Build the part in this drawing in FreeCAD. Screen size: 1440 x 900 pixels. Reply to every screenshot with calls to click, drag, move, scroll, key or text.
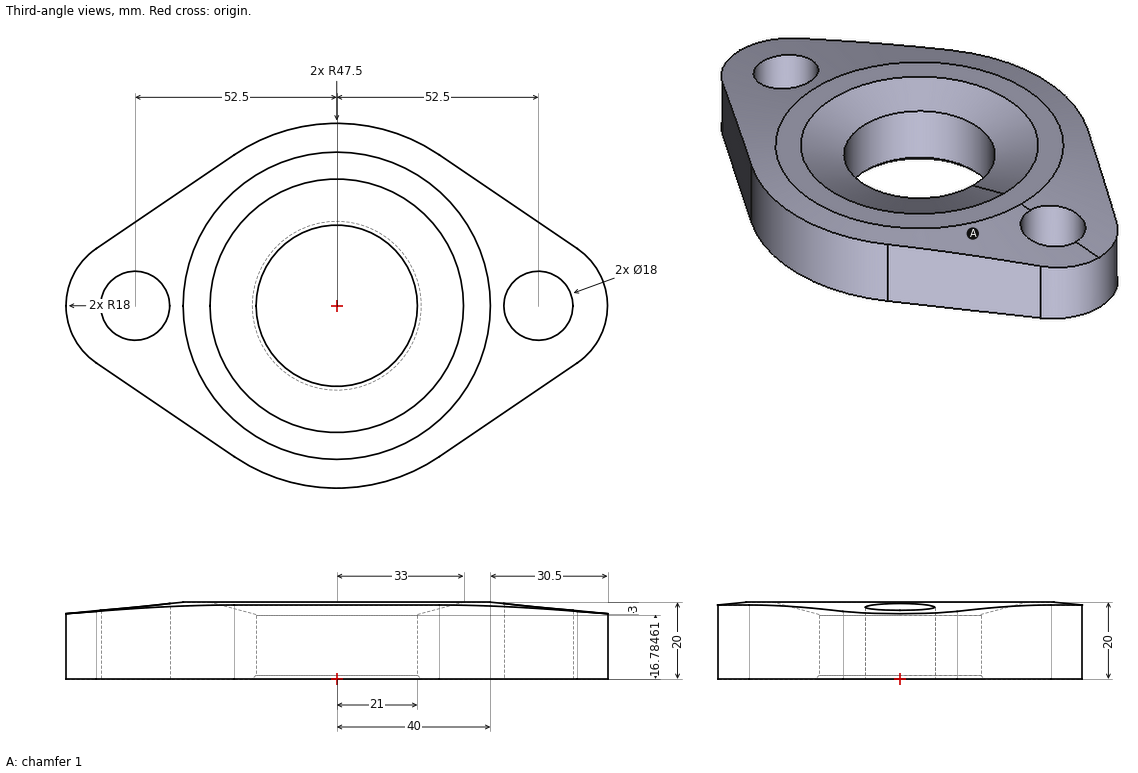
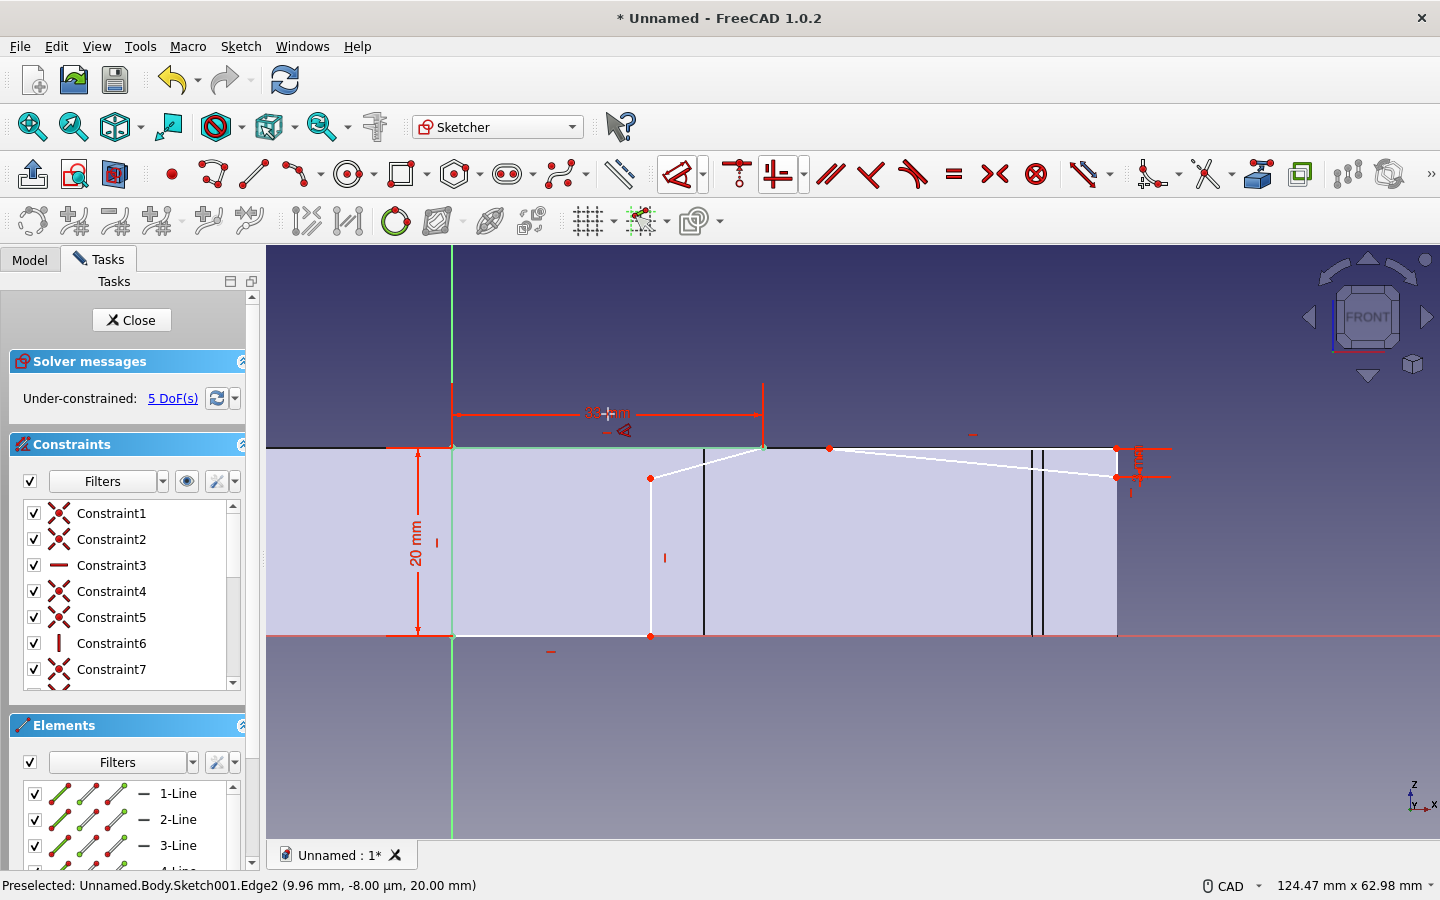
click(591, 636)
click(551, 670)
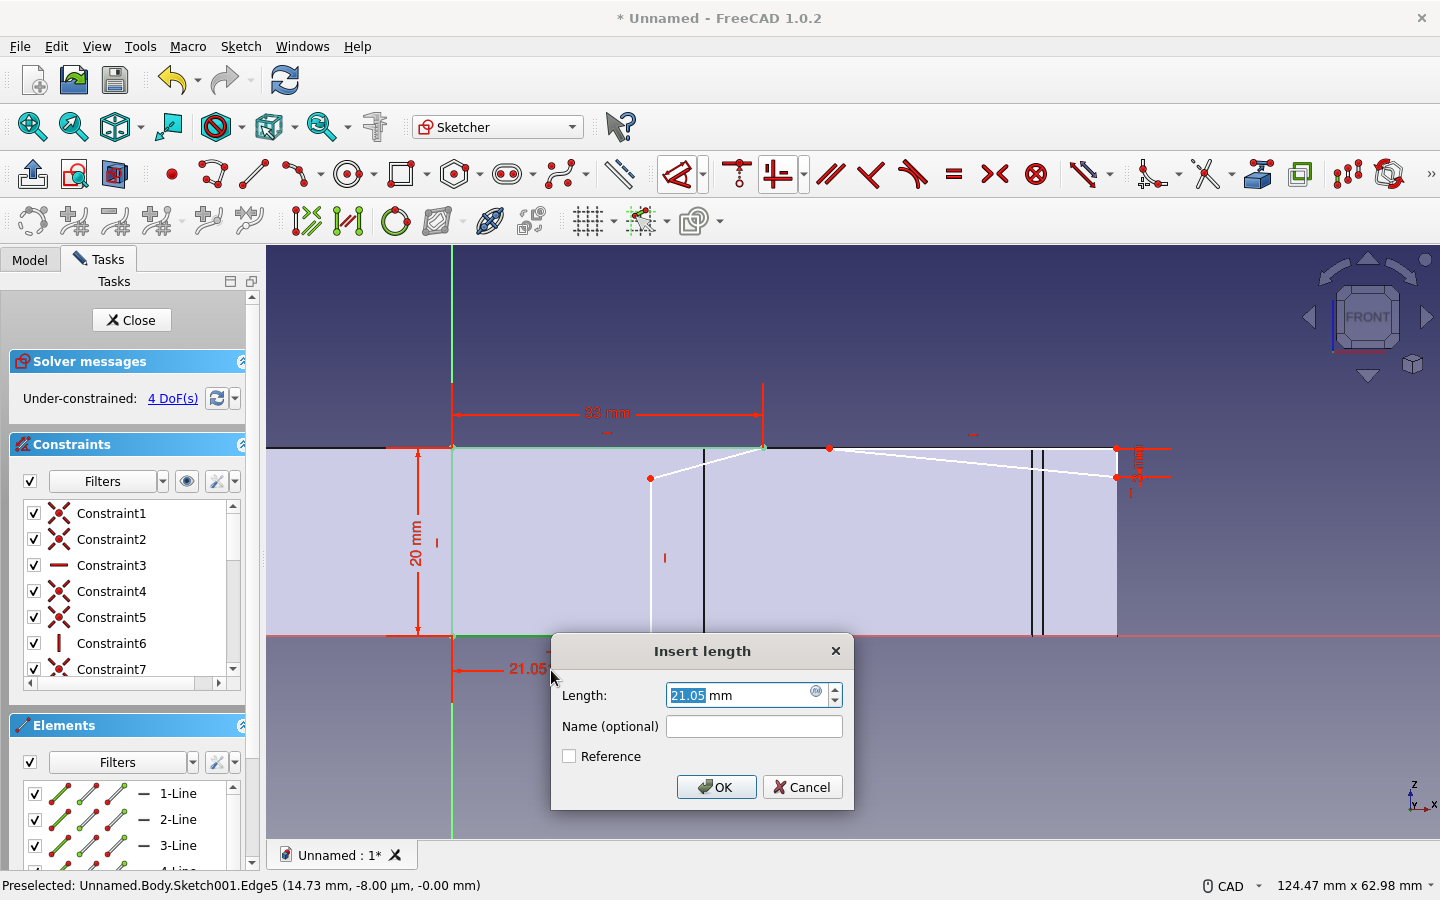
text(21)
key(Return)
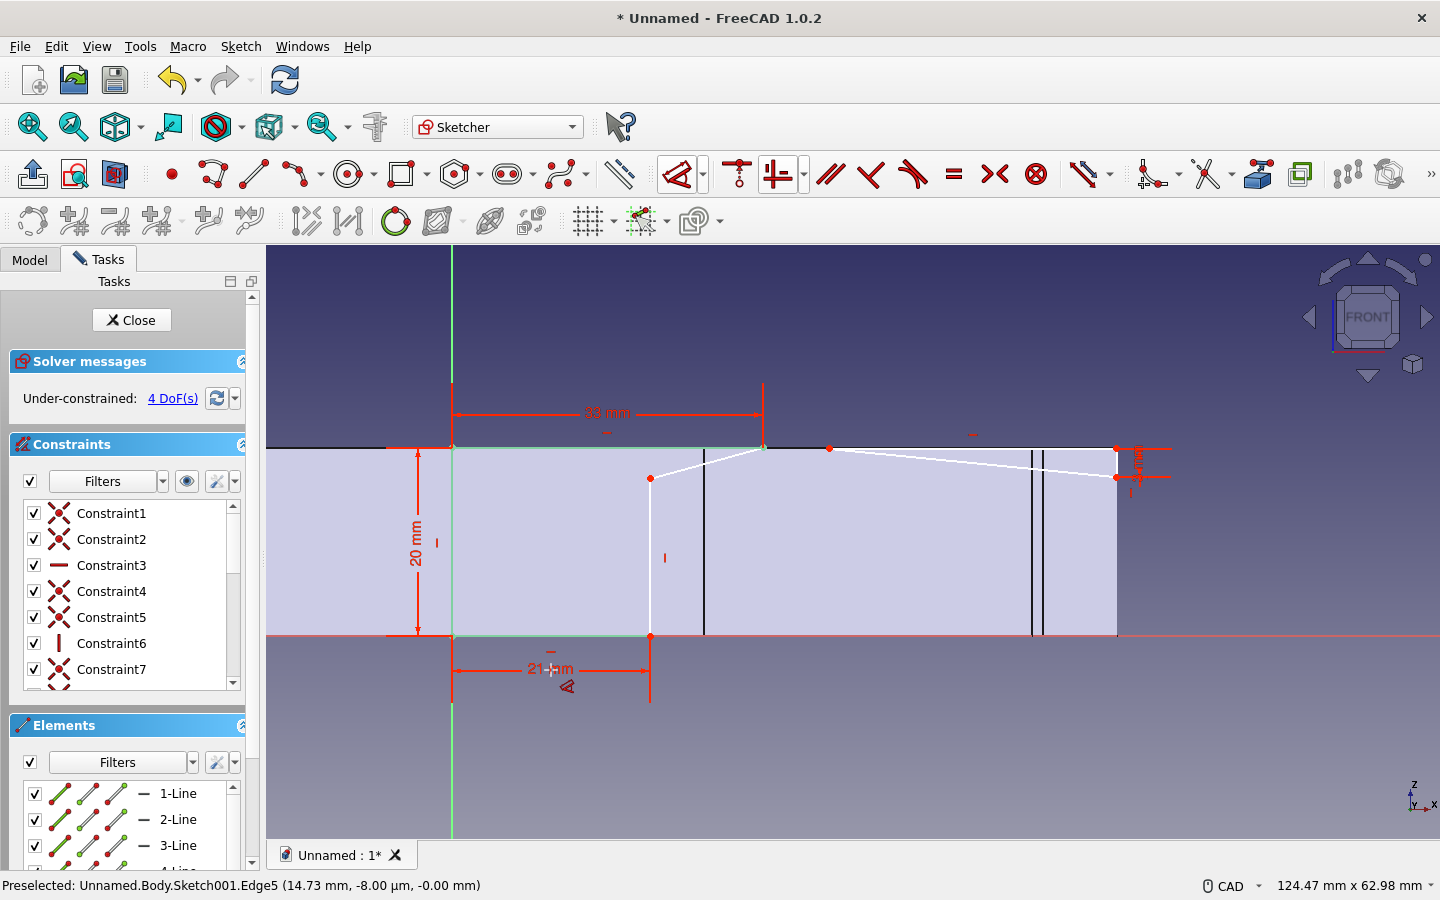
click(830, 449)
click(641, 670)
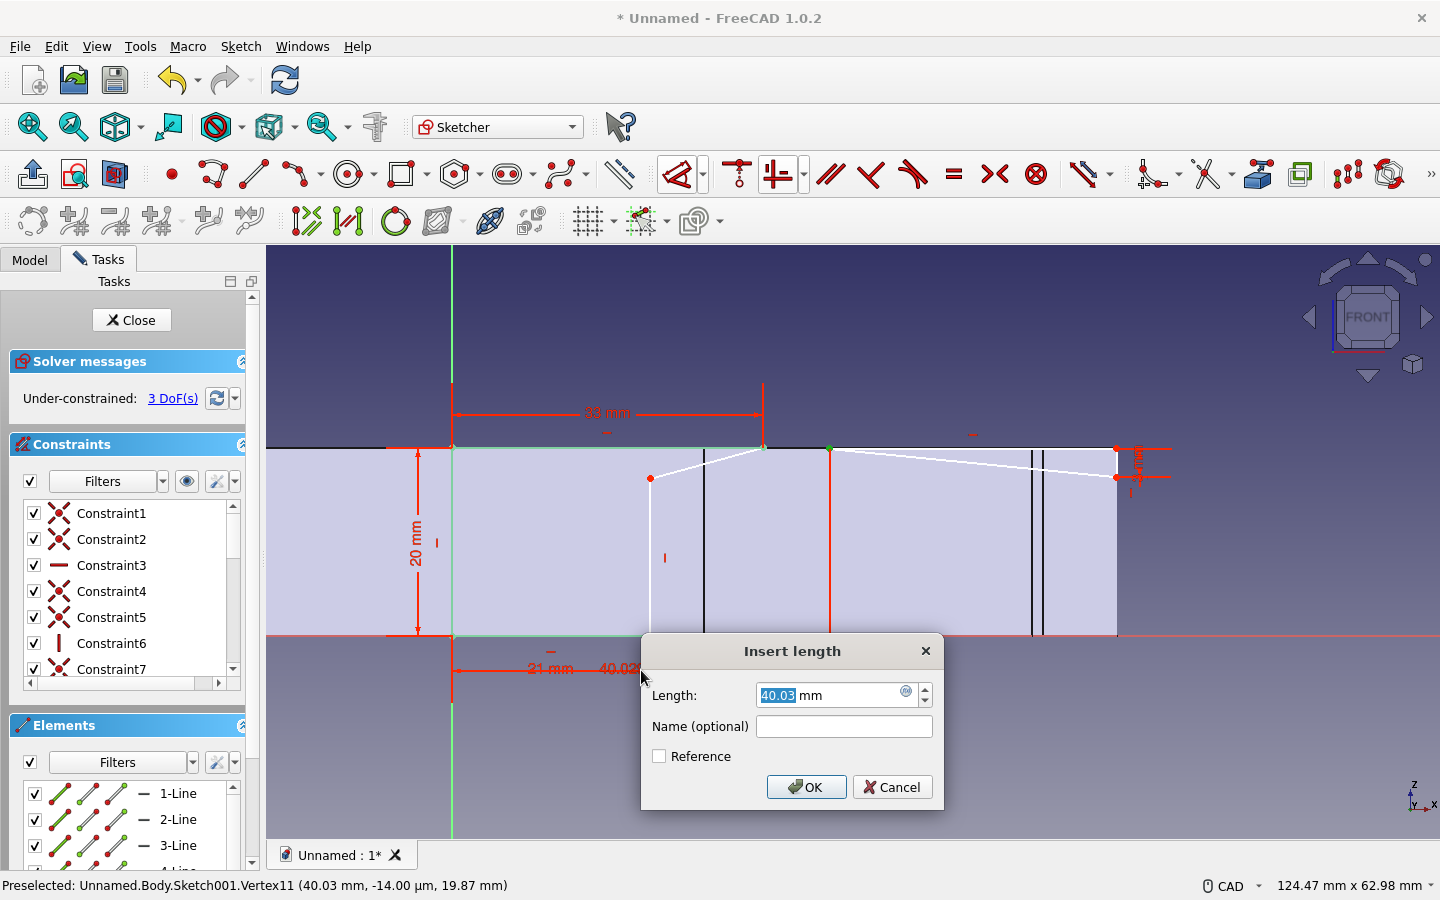
text(40)
key(Return)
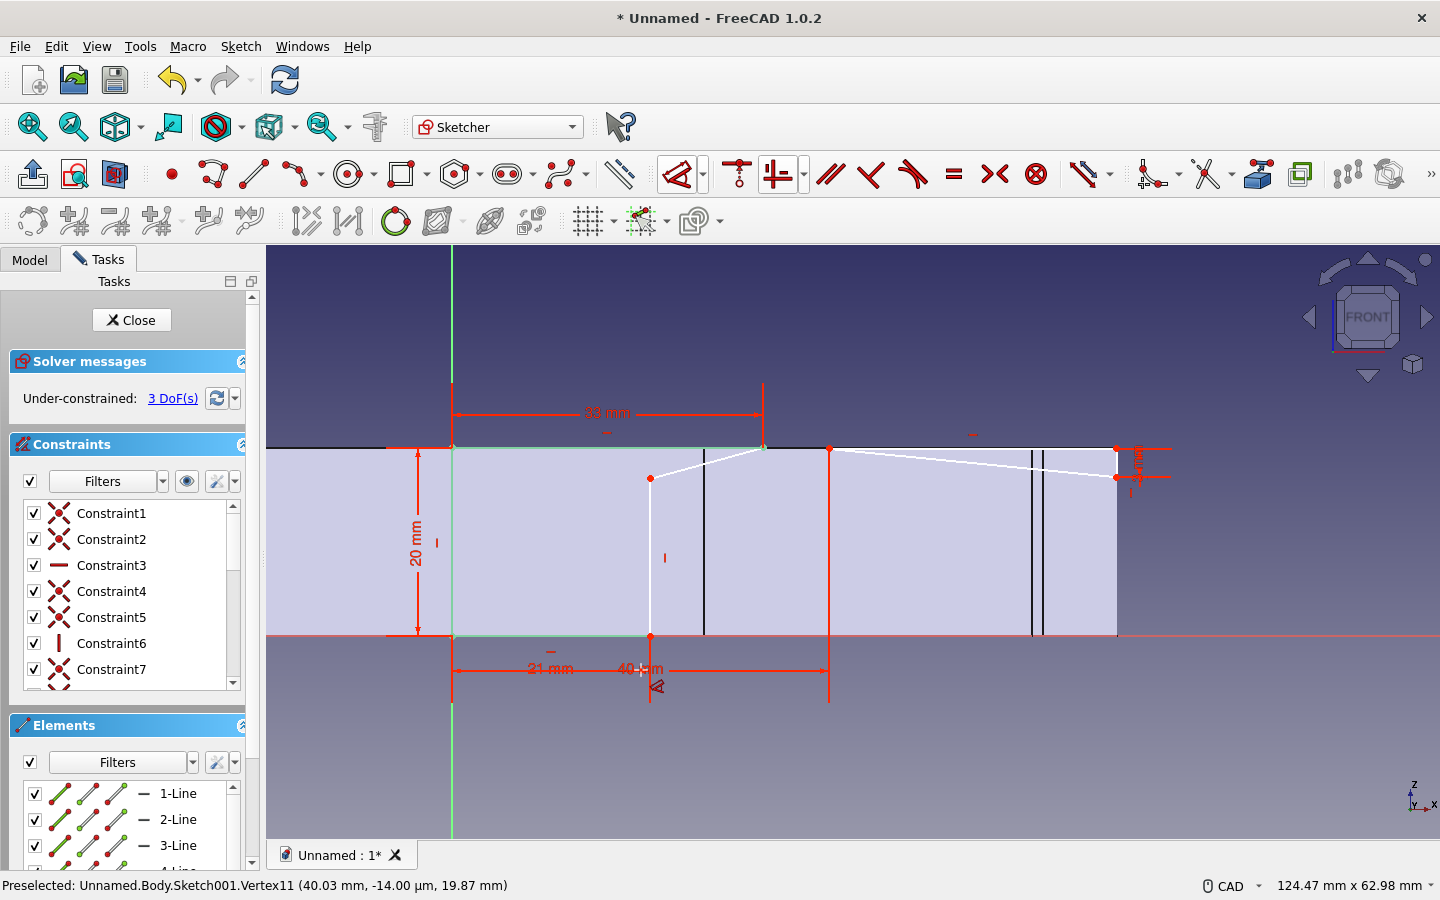
click(829, 449)
click(418, 500)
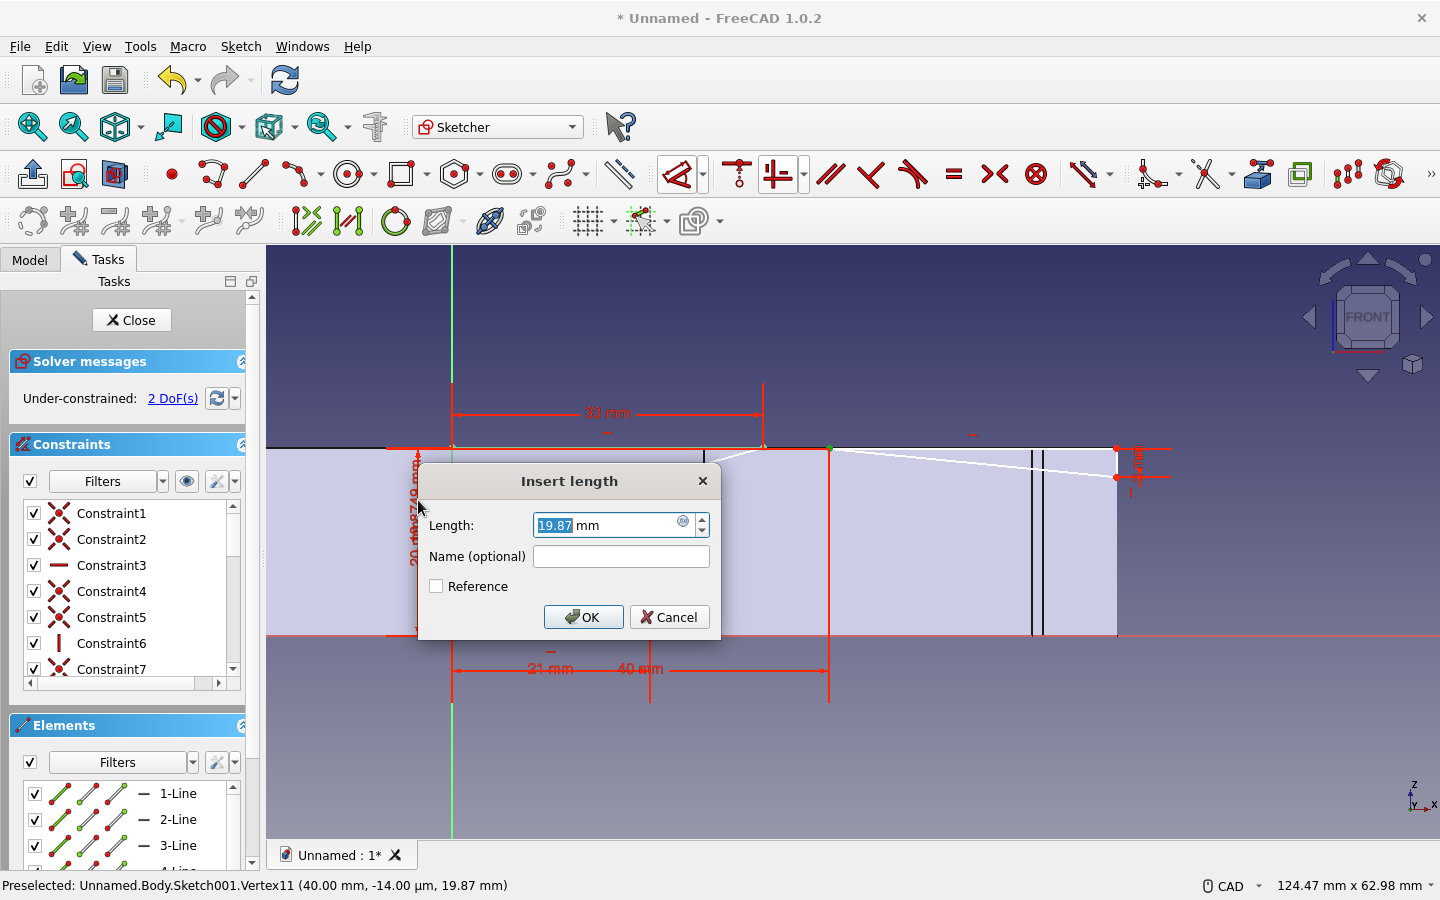
text(20)
key(Return)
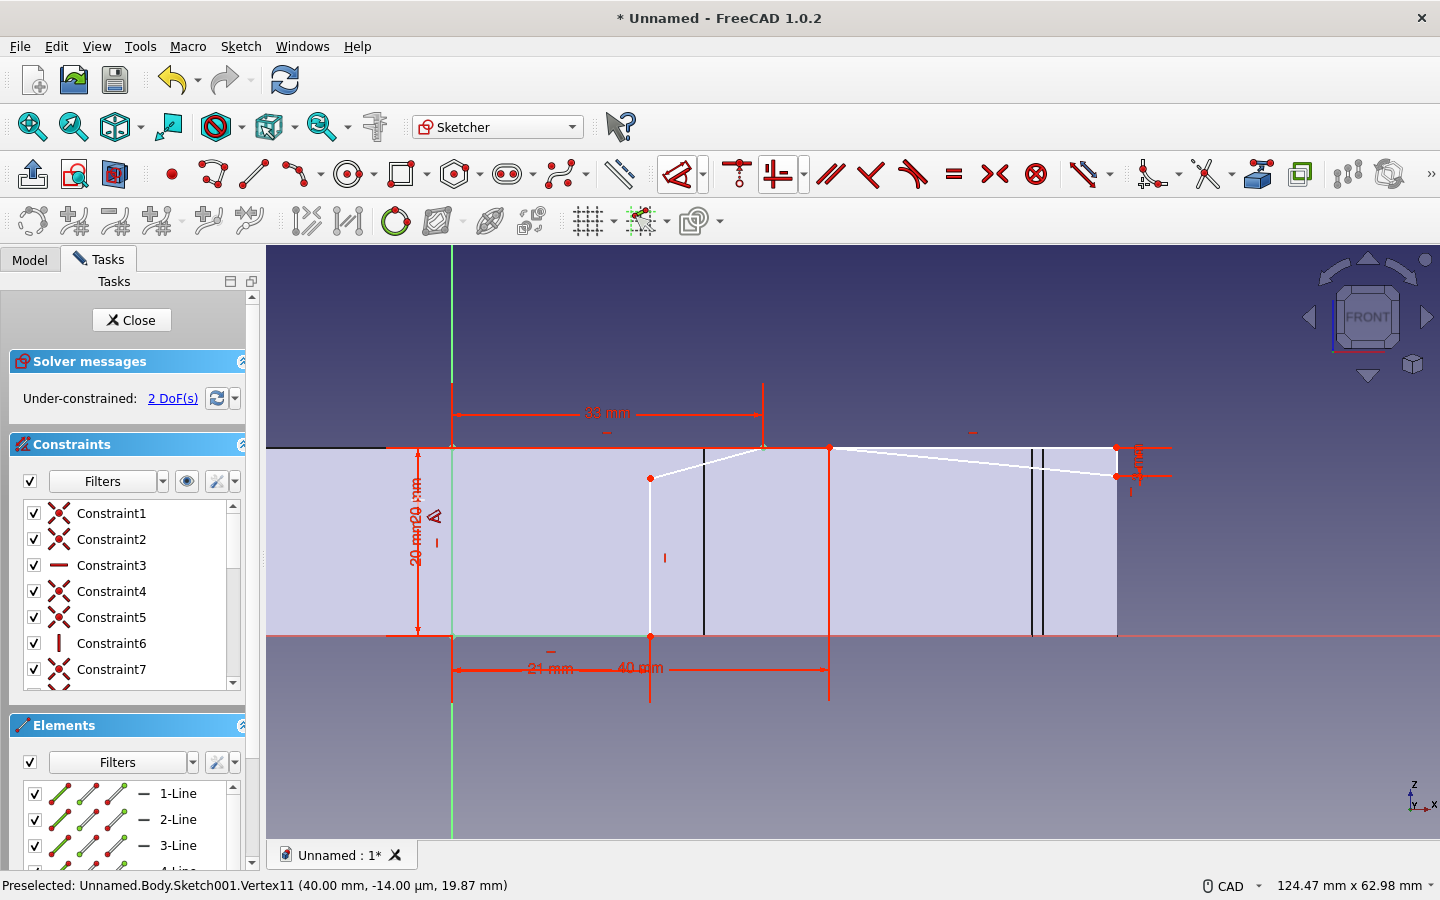
click(1030, 448)
click(973, 414)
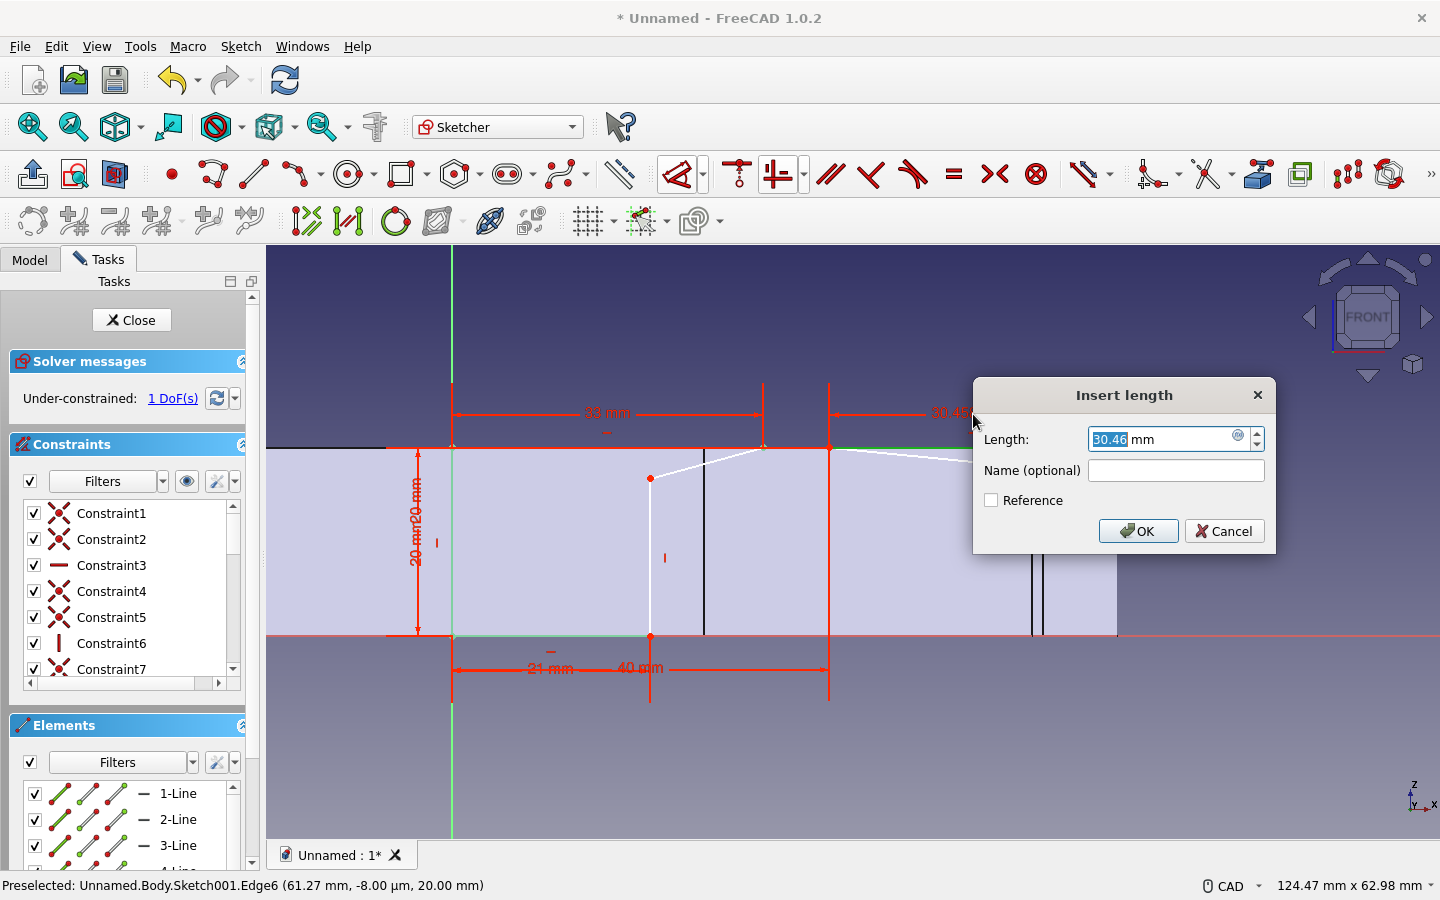
text(30.5)
key(Return)